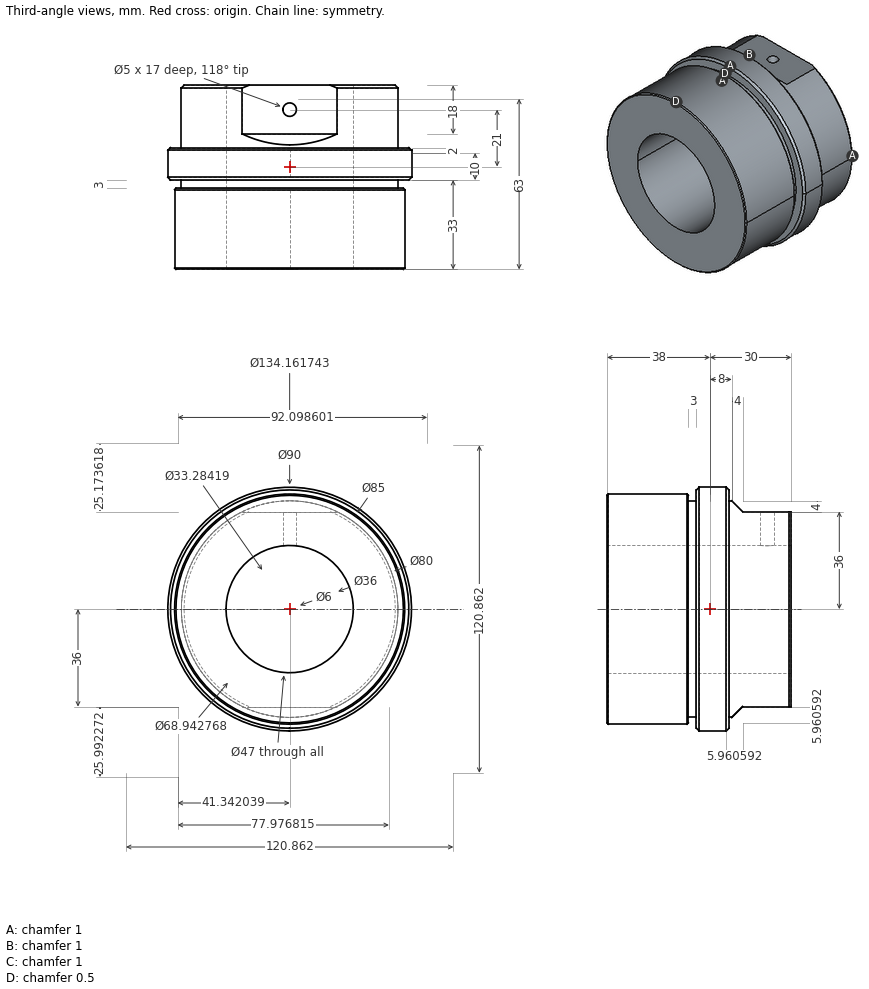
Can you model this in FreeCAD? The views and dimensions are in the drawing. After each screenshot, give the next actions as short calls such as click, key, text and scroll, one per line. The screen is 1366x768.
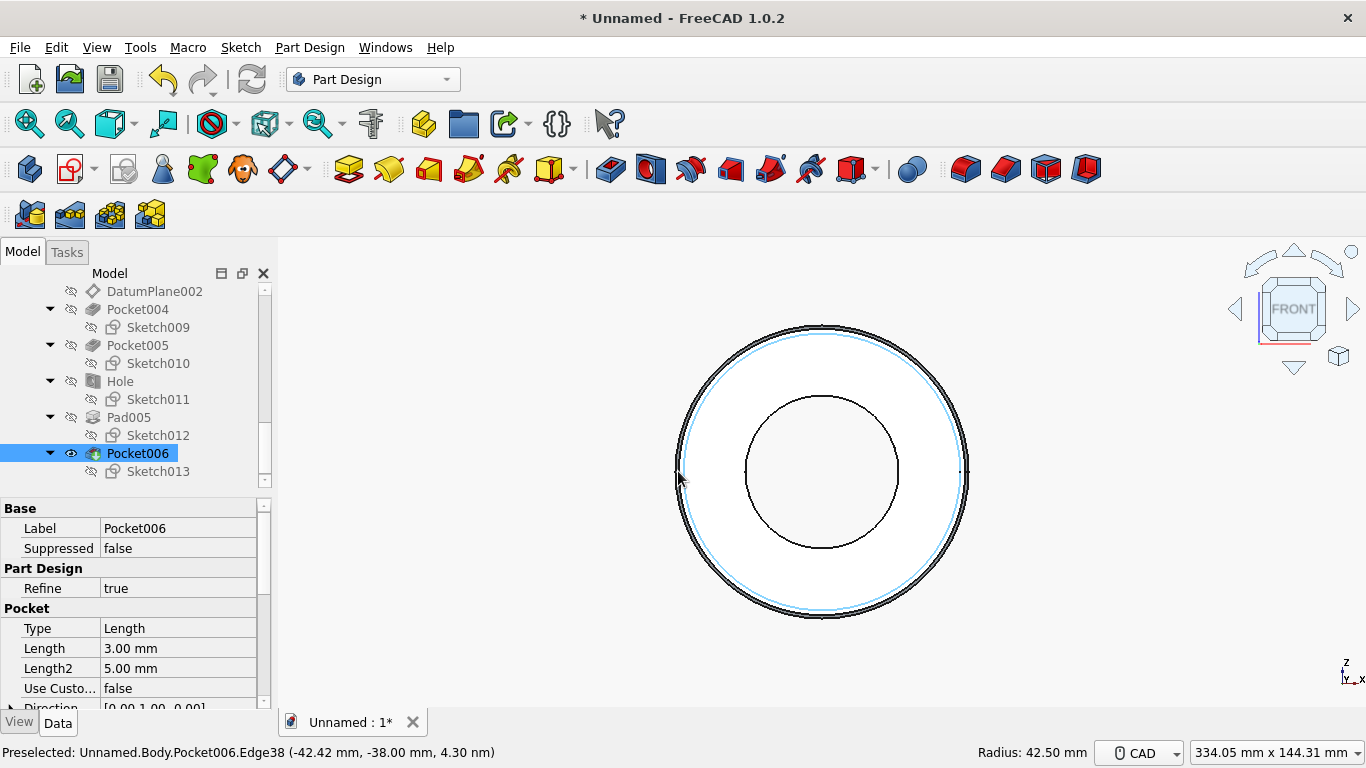
key(0)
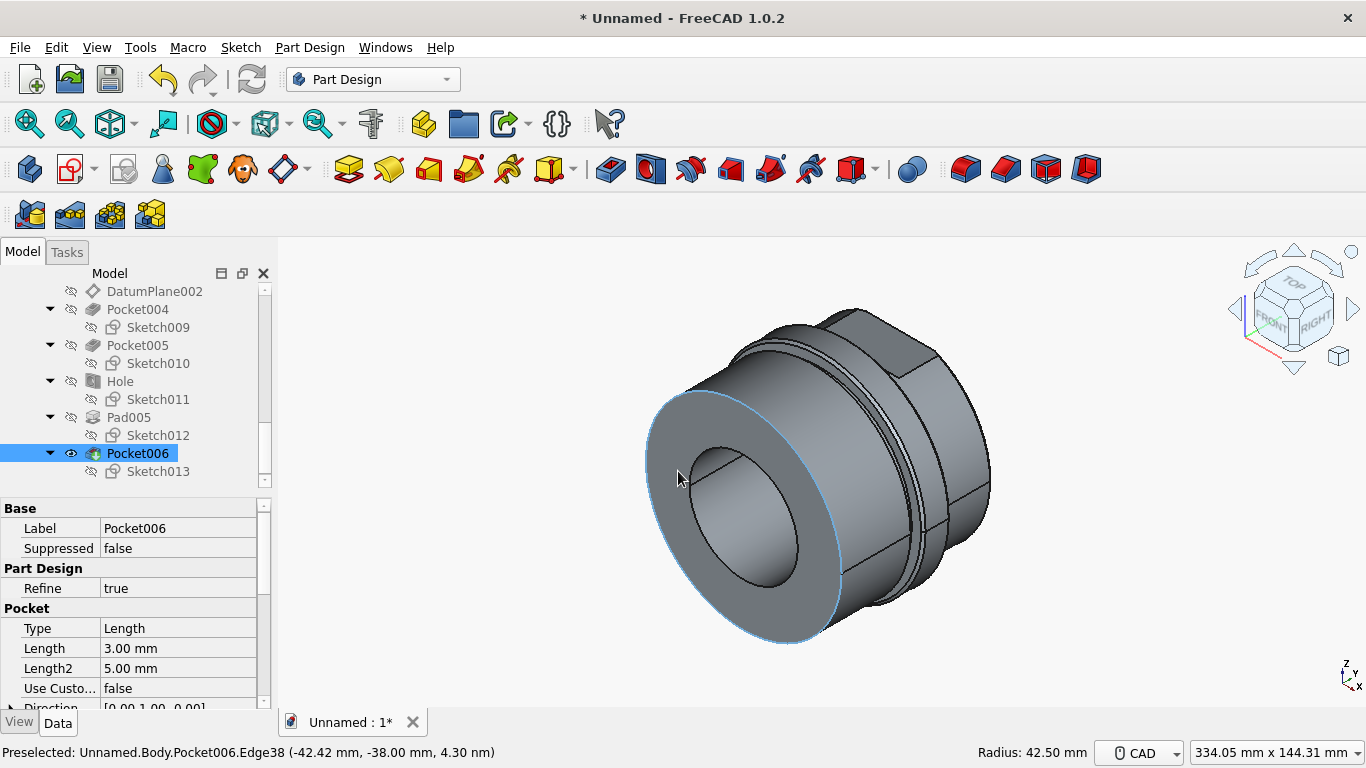
click(843, 386, ctrl)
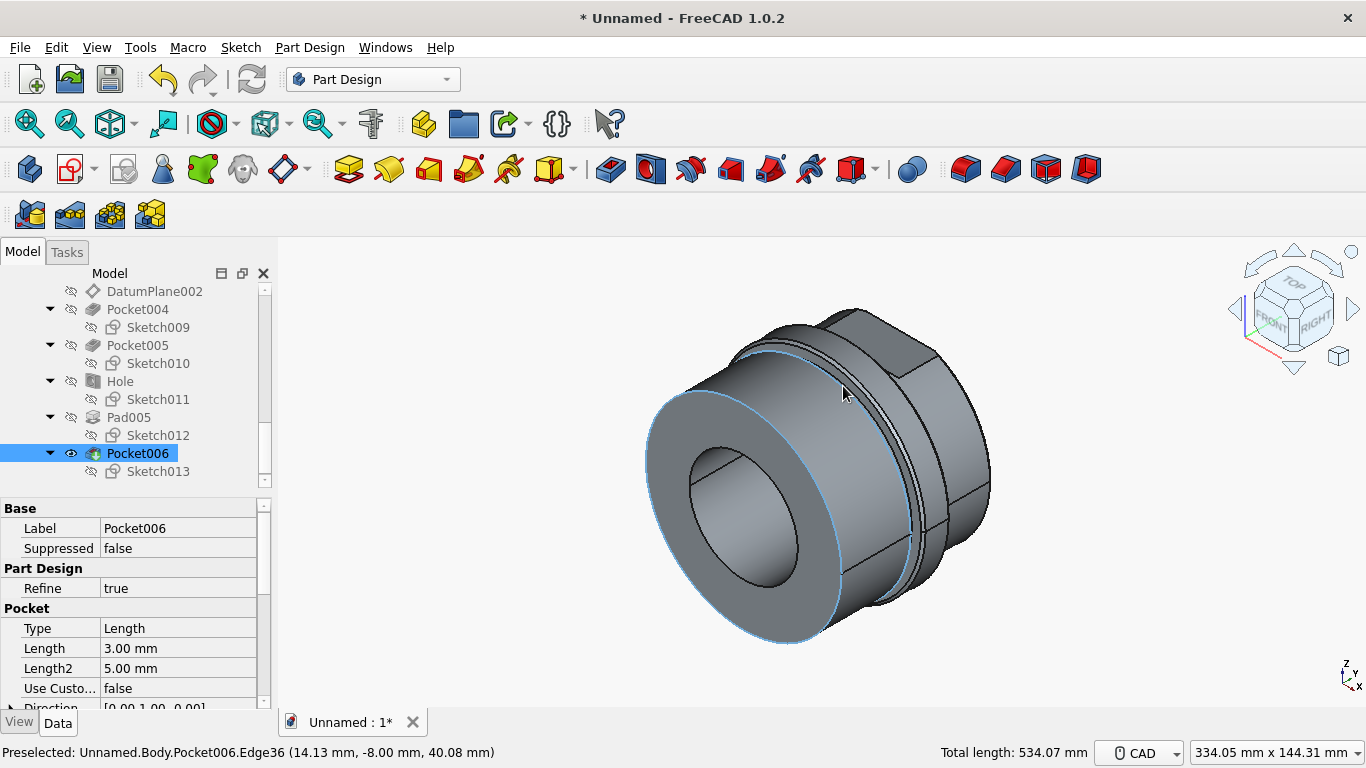
click(1006, 170)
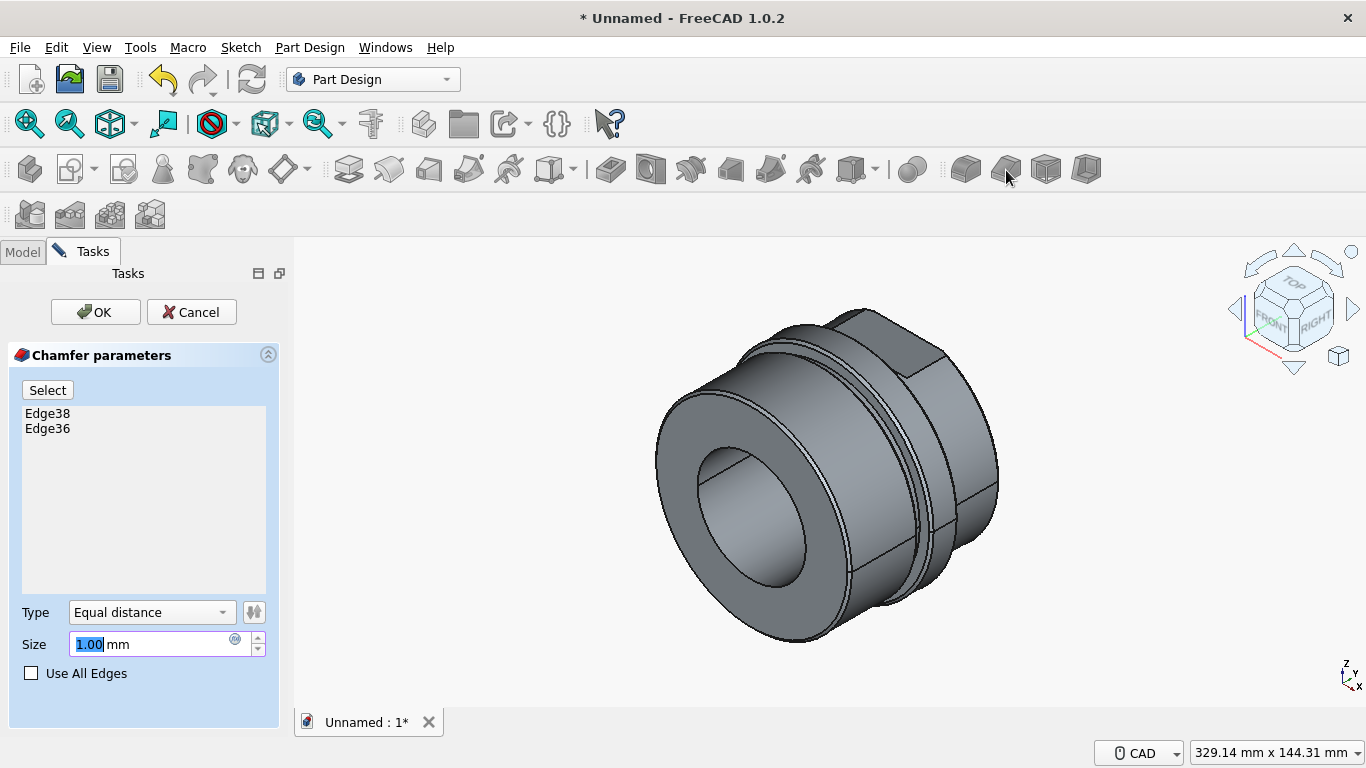
text(0.5)
key(Tab)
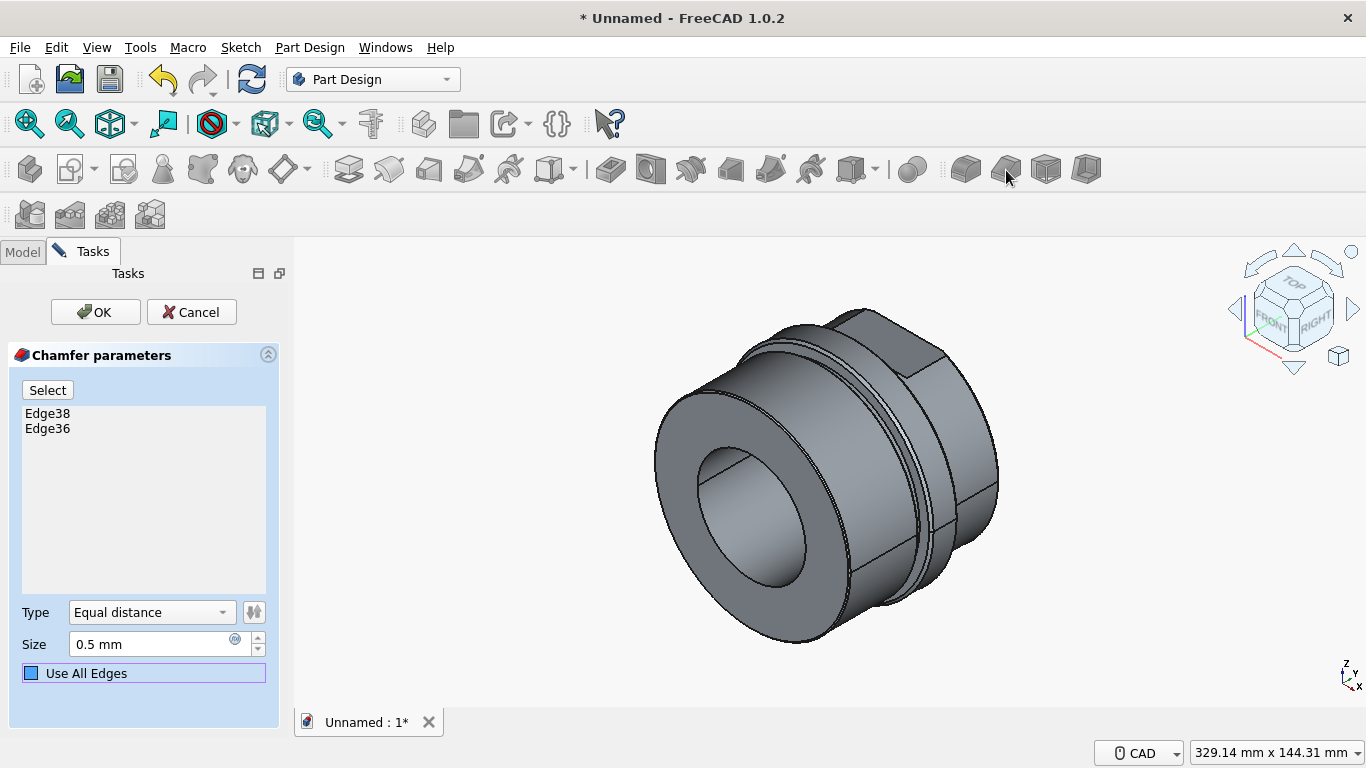
click(96, 312)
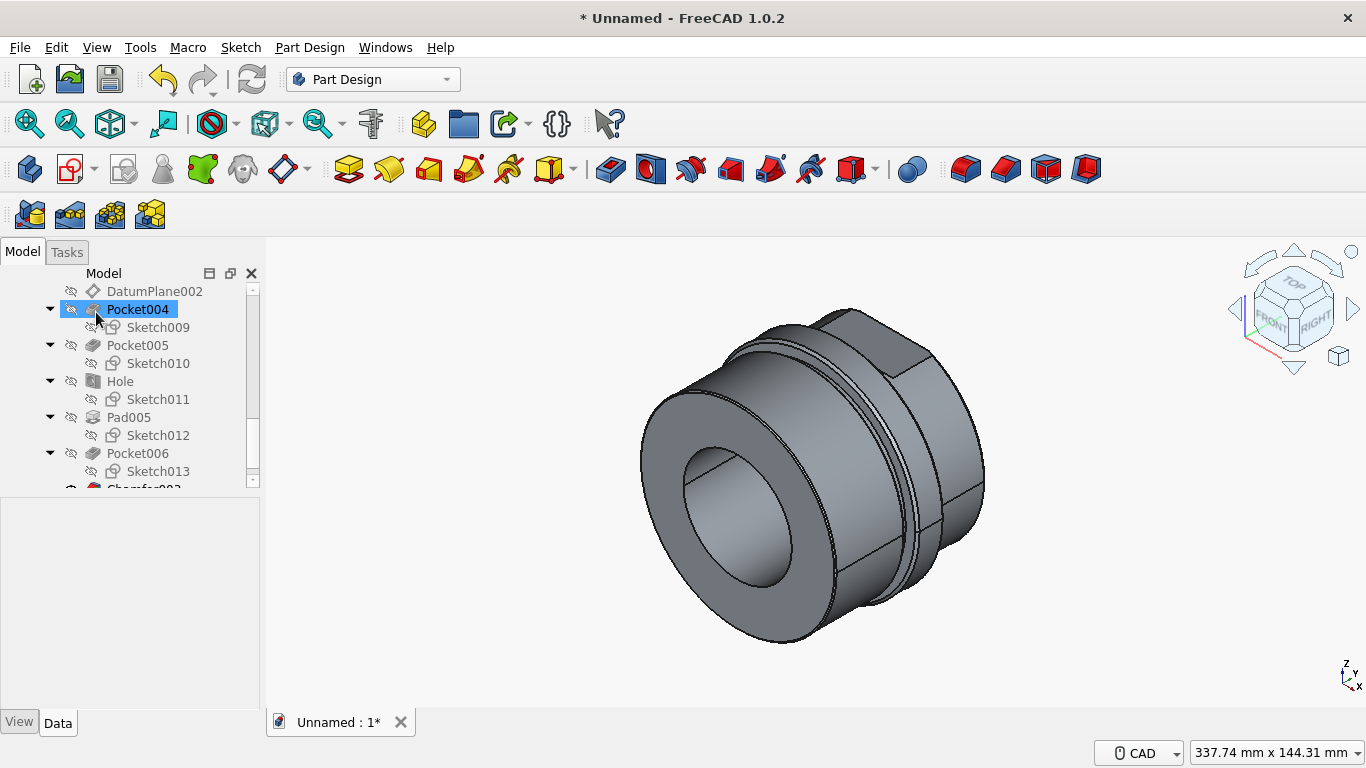
click(885, 349)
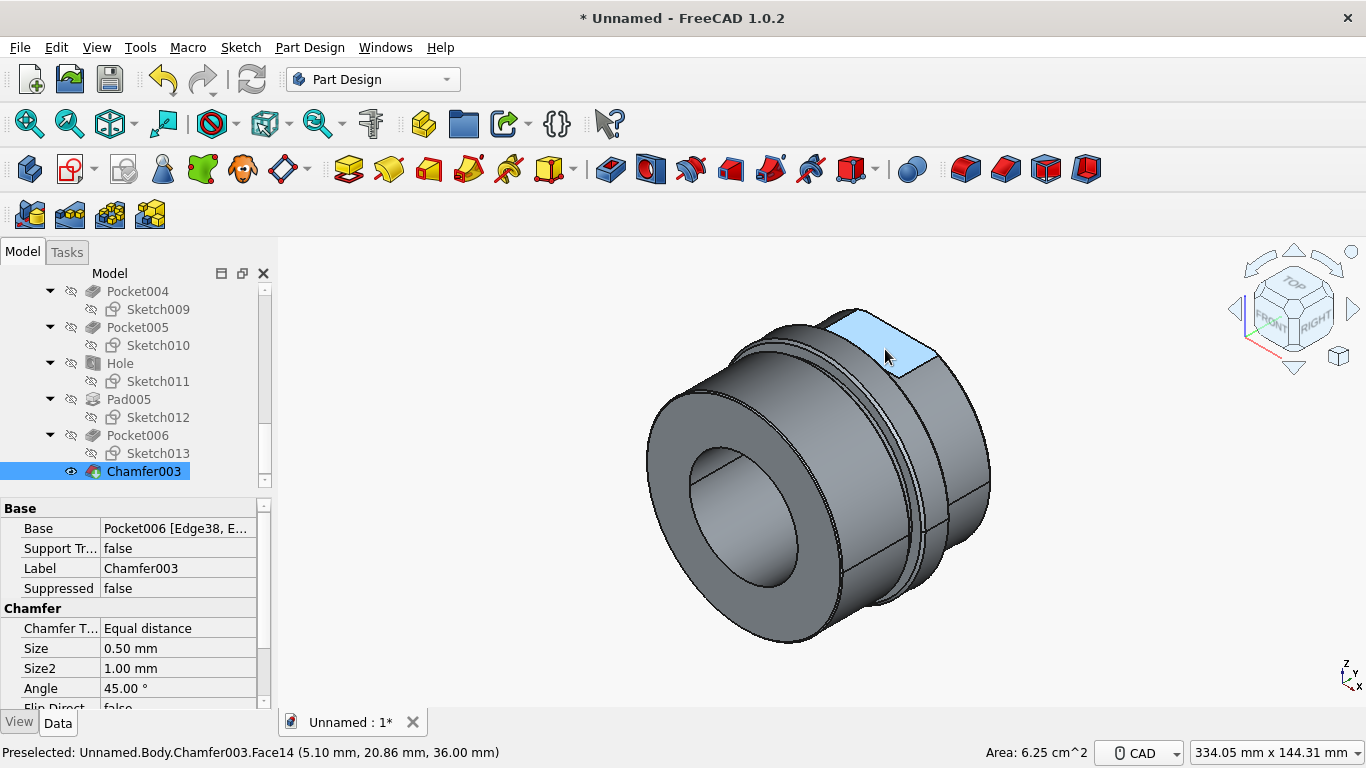
click(70, 170)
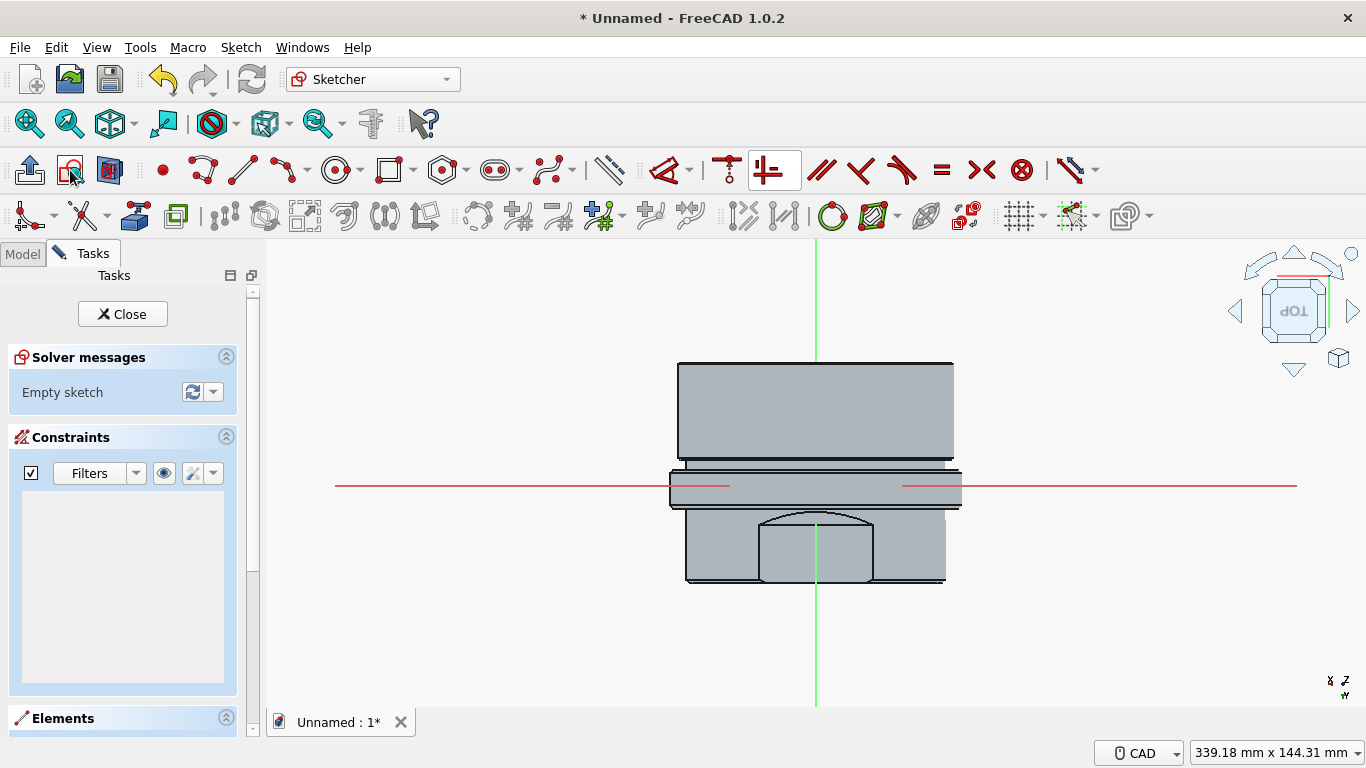
scroll(820, 559, up, 14)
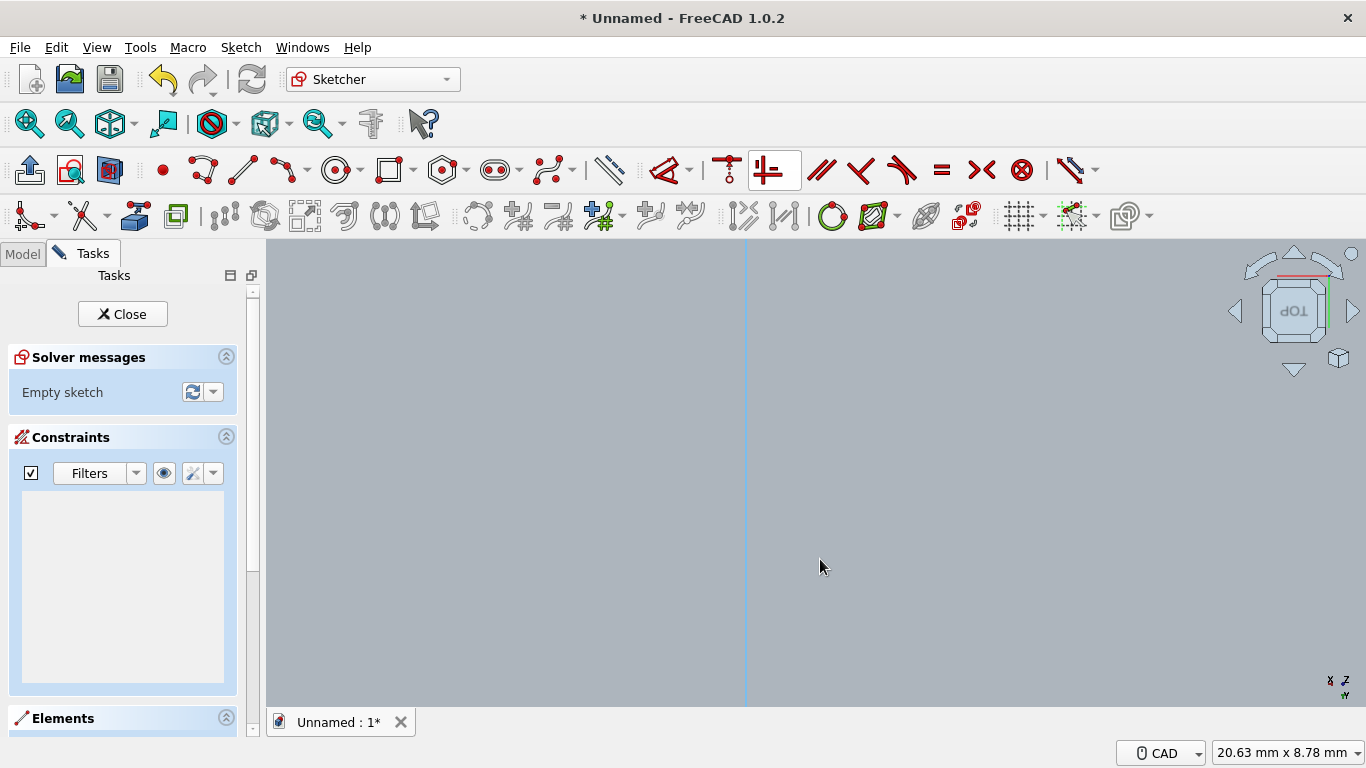
click(336, 170)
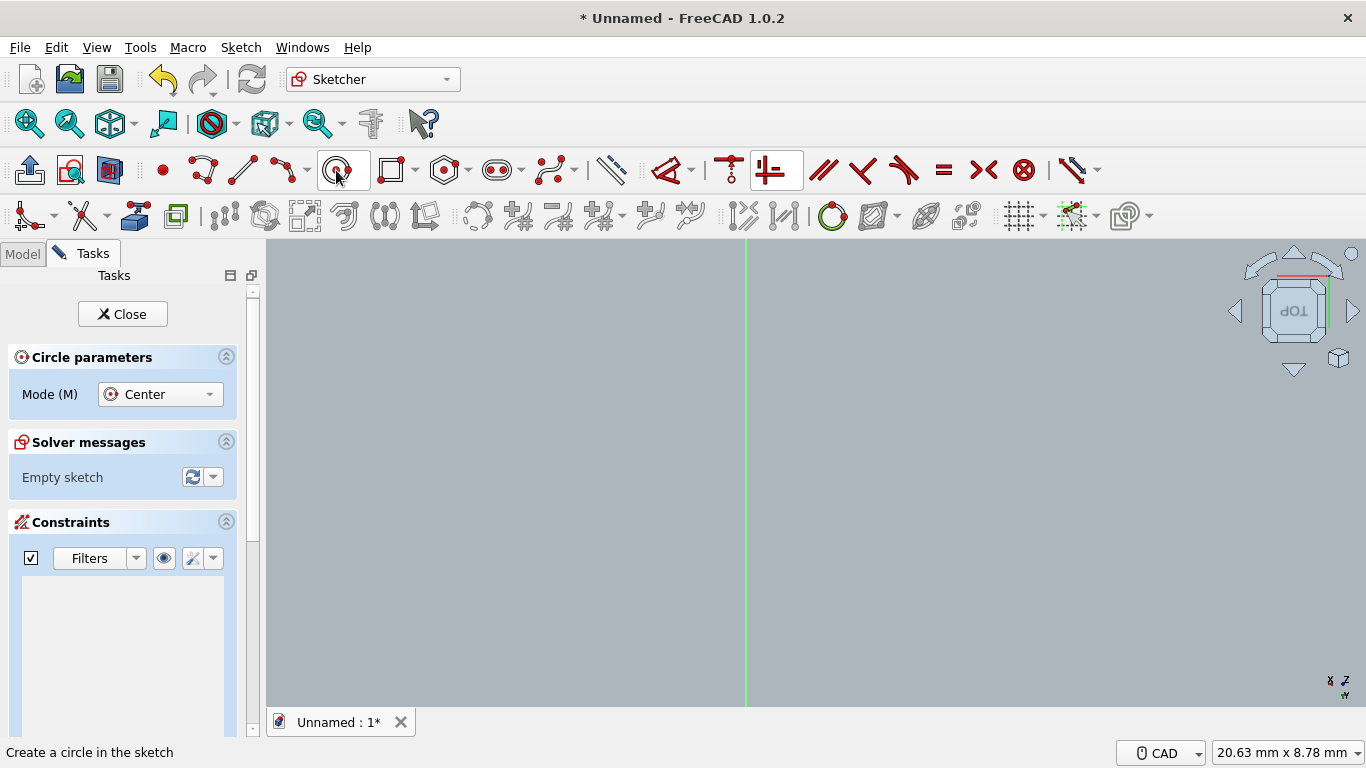
click(746, 467)
click(841, 373)
key(Escape)